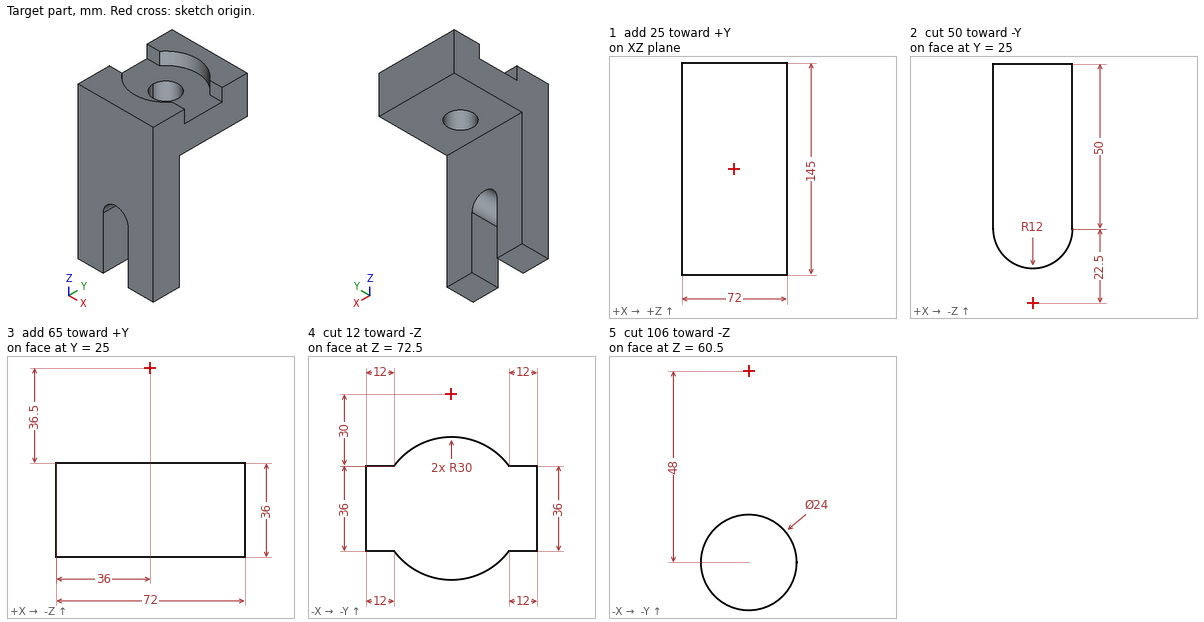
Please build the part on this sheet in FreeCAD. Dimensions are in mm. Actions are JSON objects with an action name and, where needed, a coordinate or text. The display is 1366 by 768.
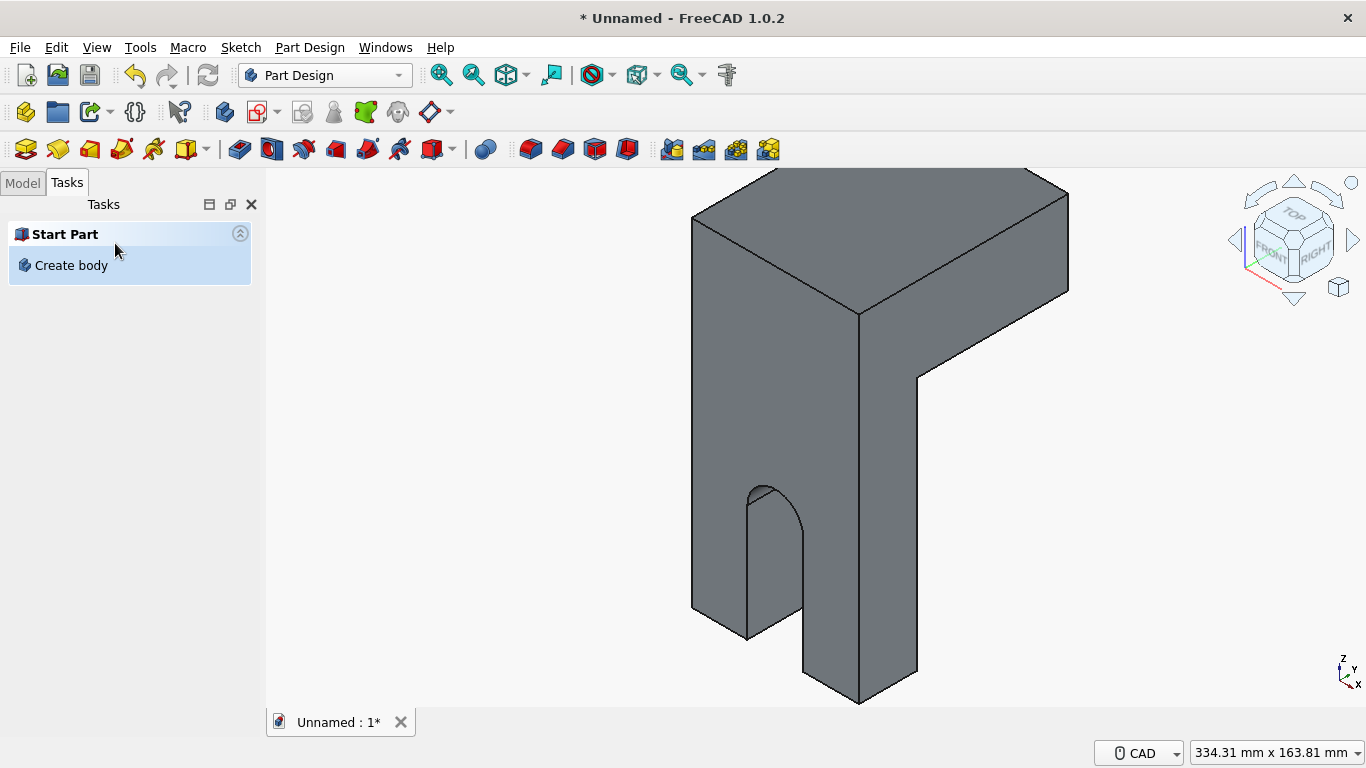
{"action": "left_click", "coordinate": [442, 76]}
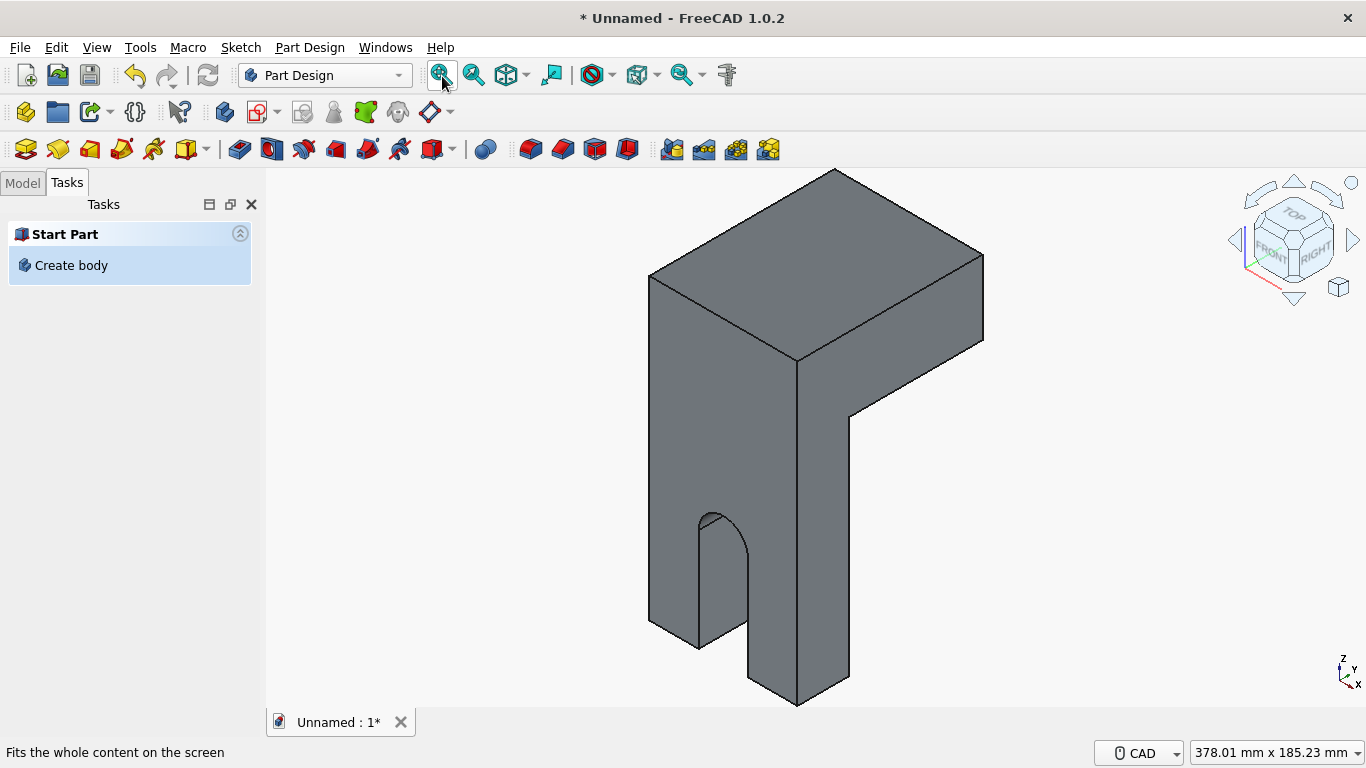
{"action": "left_click", "coordinate": [816, 264]}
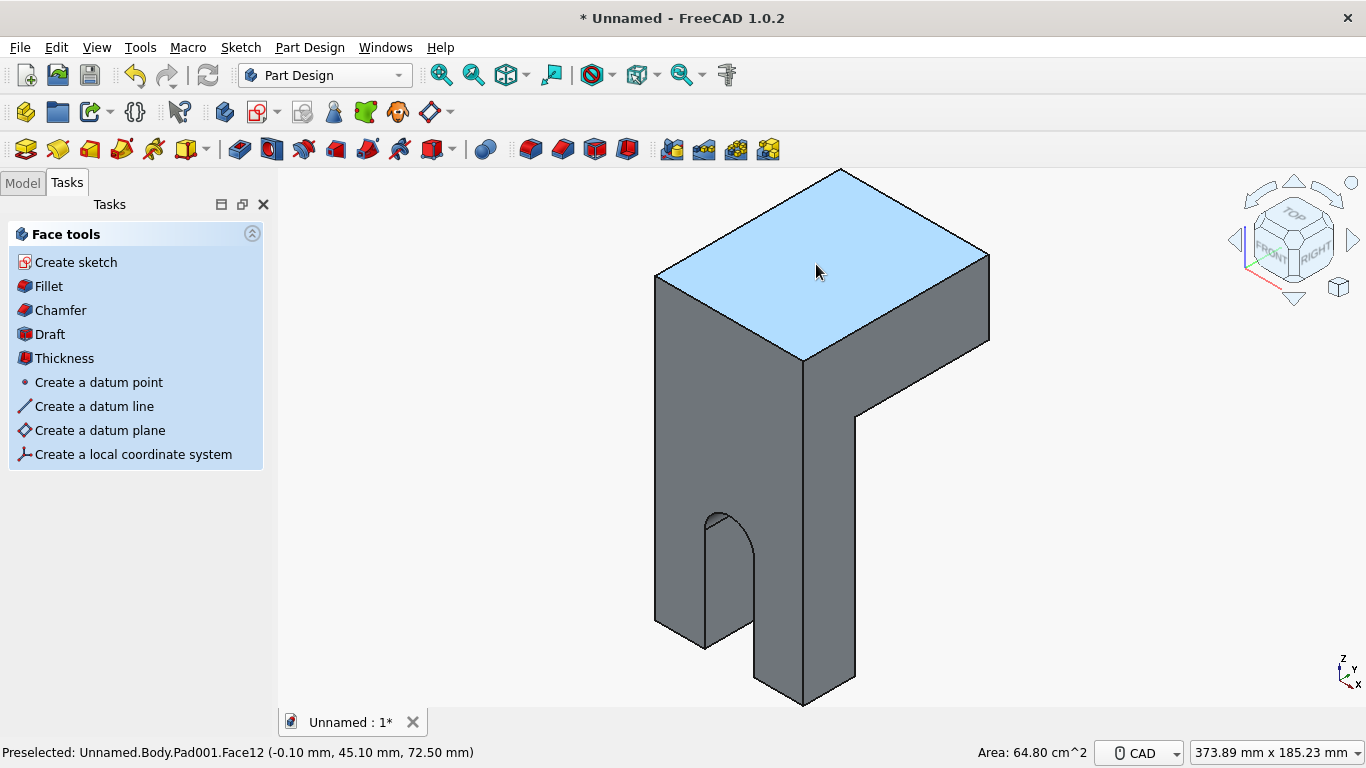
{"action": "left_click", "coordinate": [258, 112]}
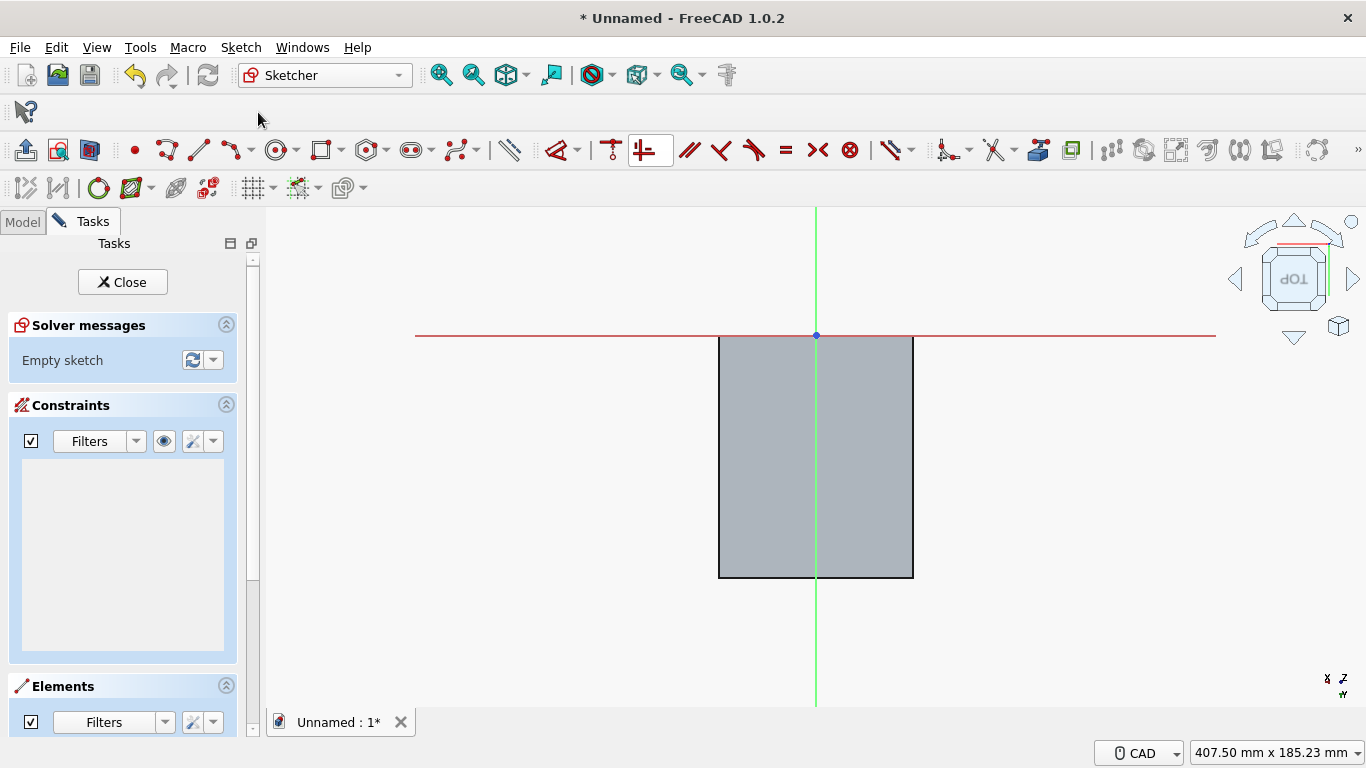
{"action": "scroll", "coordinate": [955, 408], "scroll_direction": "up", "scroll_amount": 2}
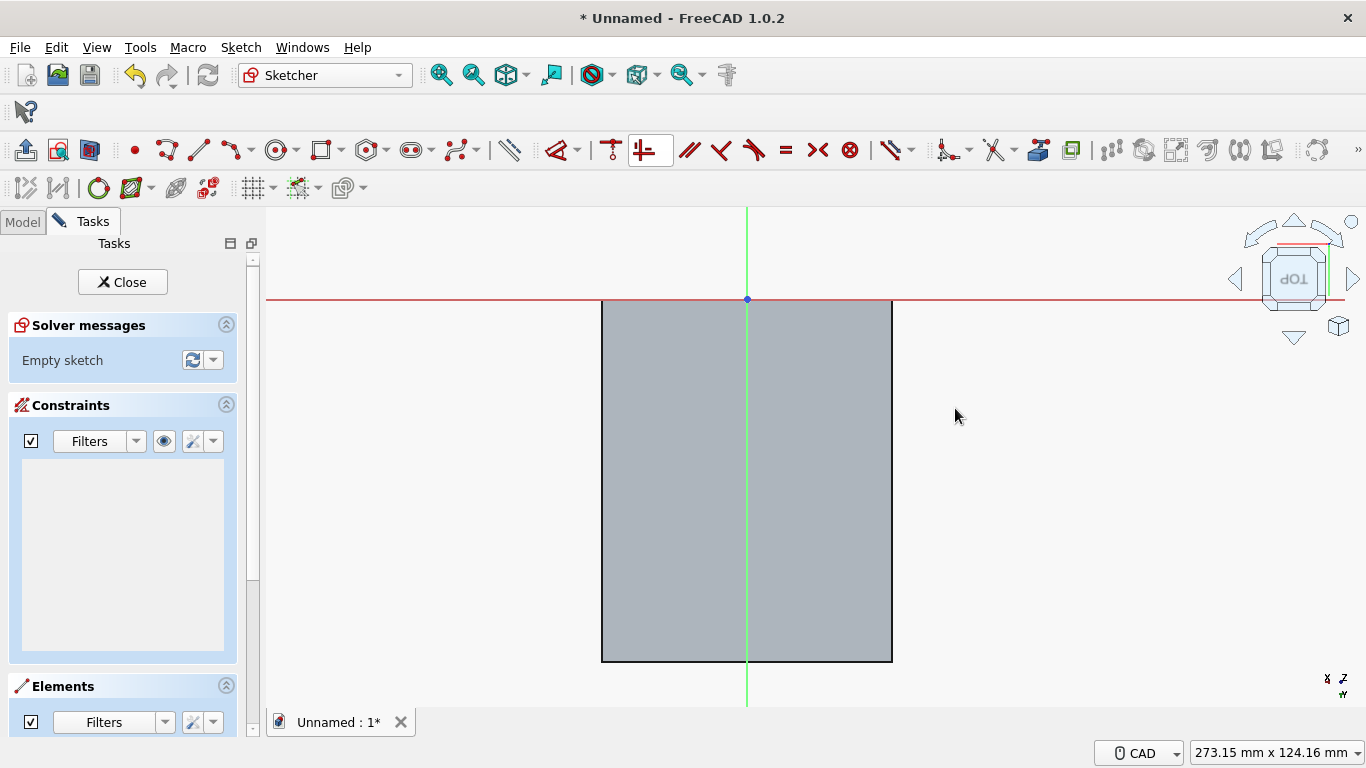
{"action": "left_click", "coordinate": [168, 150]}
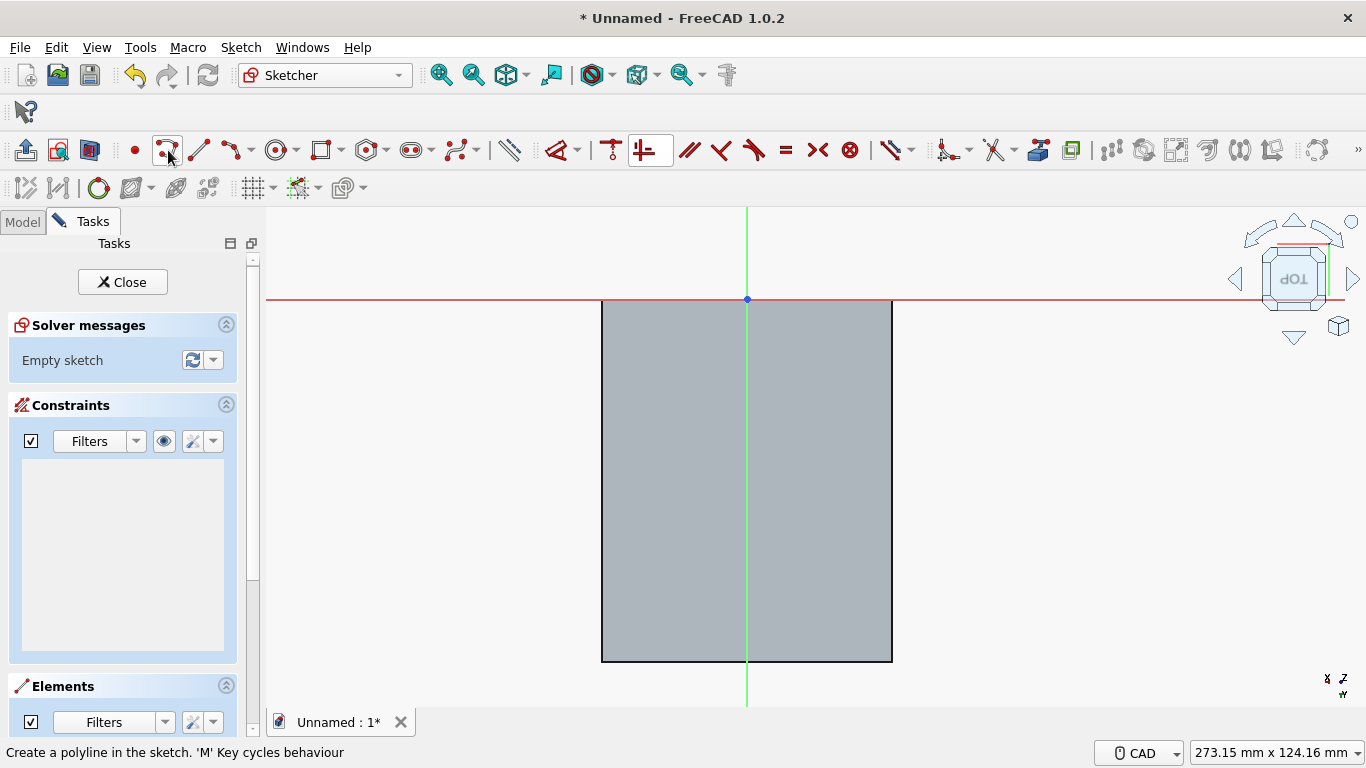
{"action": "left_click", "coordinate": [651, 420]}
{"action": "left_click", "coordinate": [602, 420]}
{"action": "left_click", "coordinate": [602, 565]}
{"action": "left_click", "coordinate": [651, 565]}
{"action": "right_click", "coordinate": [651, 565]}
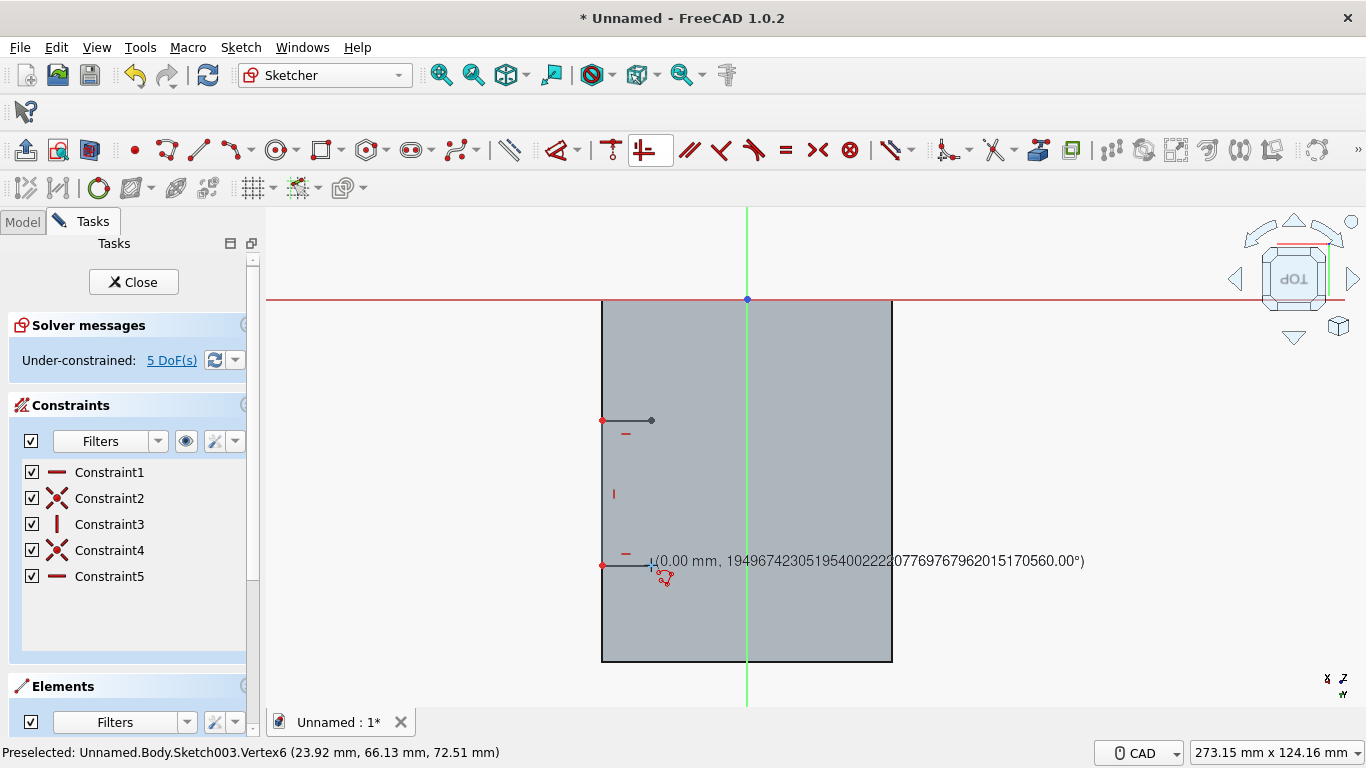
{"action": "left_click", "coordinate": [844, 565]}
{"action": "left_click", "coordinate": [892, 565]}
{"action": "left_click", "coordinate": [892, 420]}
{"action": "left_click", "coordinate": [844, 420]}
{"action": "right_click", "coordinate": [844, 420]}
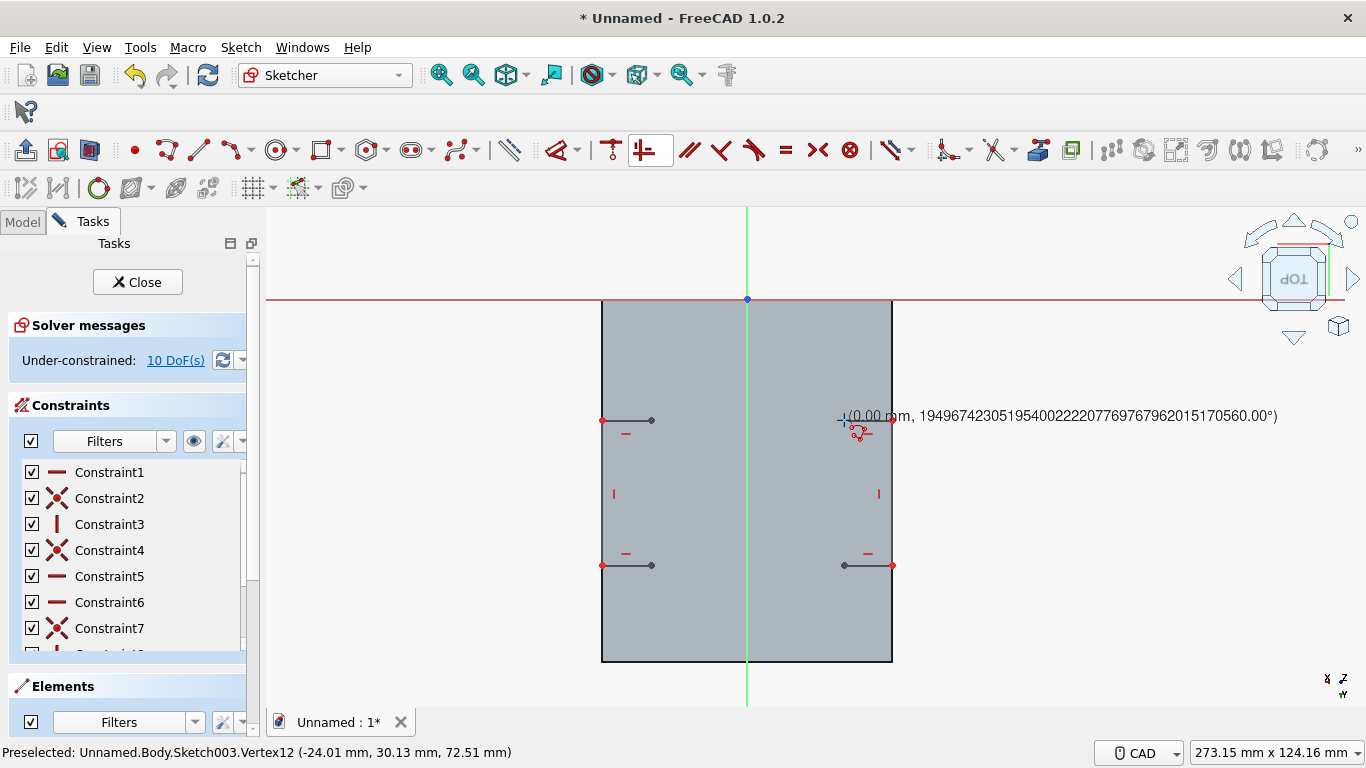
{"action": "left_click", "coordinate": [232, 150]}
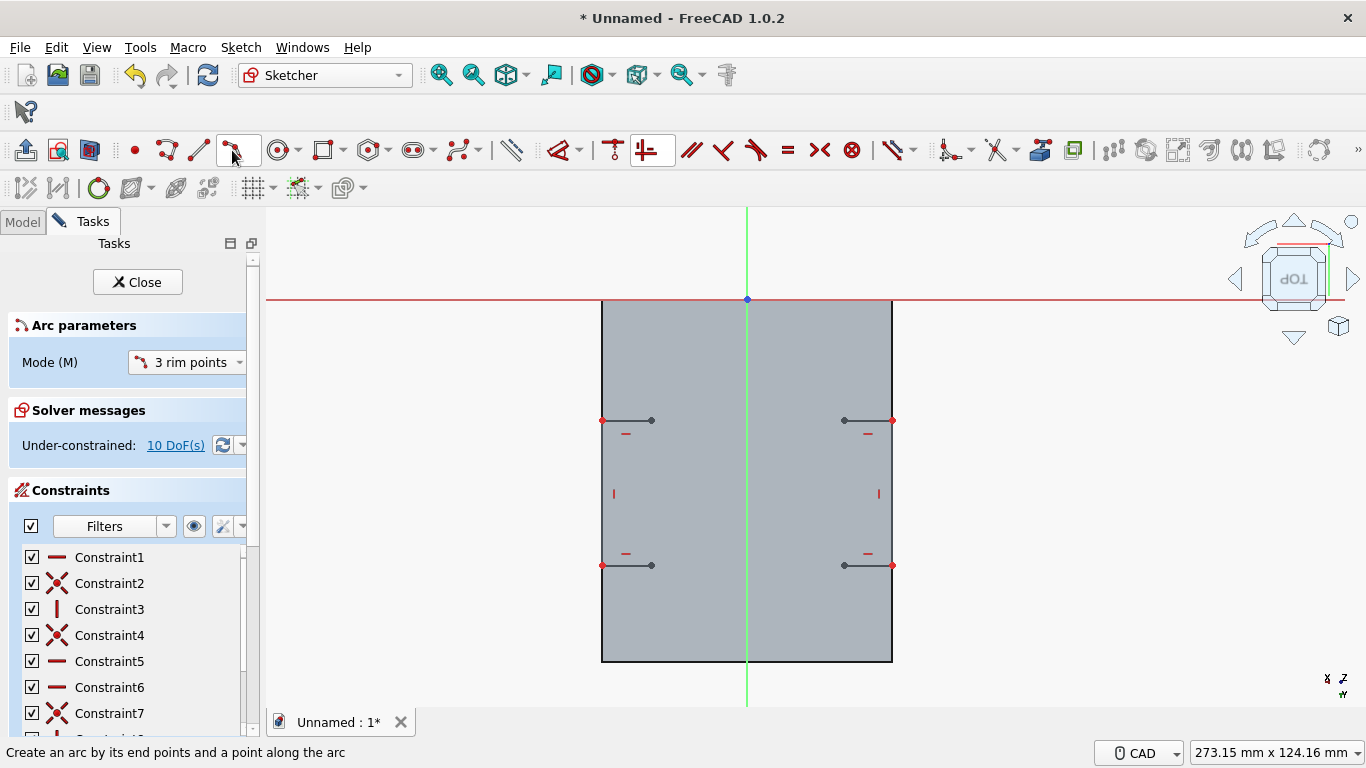
{"action": "left_click", "coordinate": [651, 566]}
{"action": "left_click", "coordinate": [844, 566]}
{"action": "left_click", "coordinate": [725, 612]}